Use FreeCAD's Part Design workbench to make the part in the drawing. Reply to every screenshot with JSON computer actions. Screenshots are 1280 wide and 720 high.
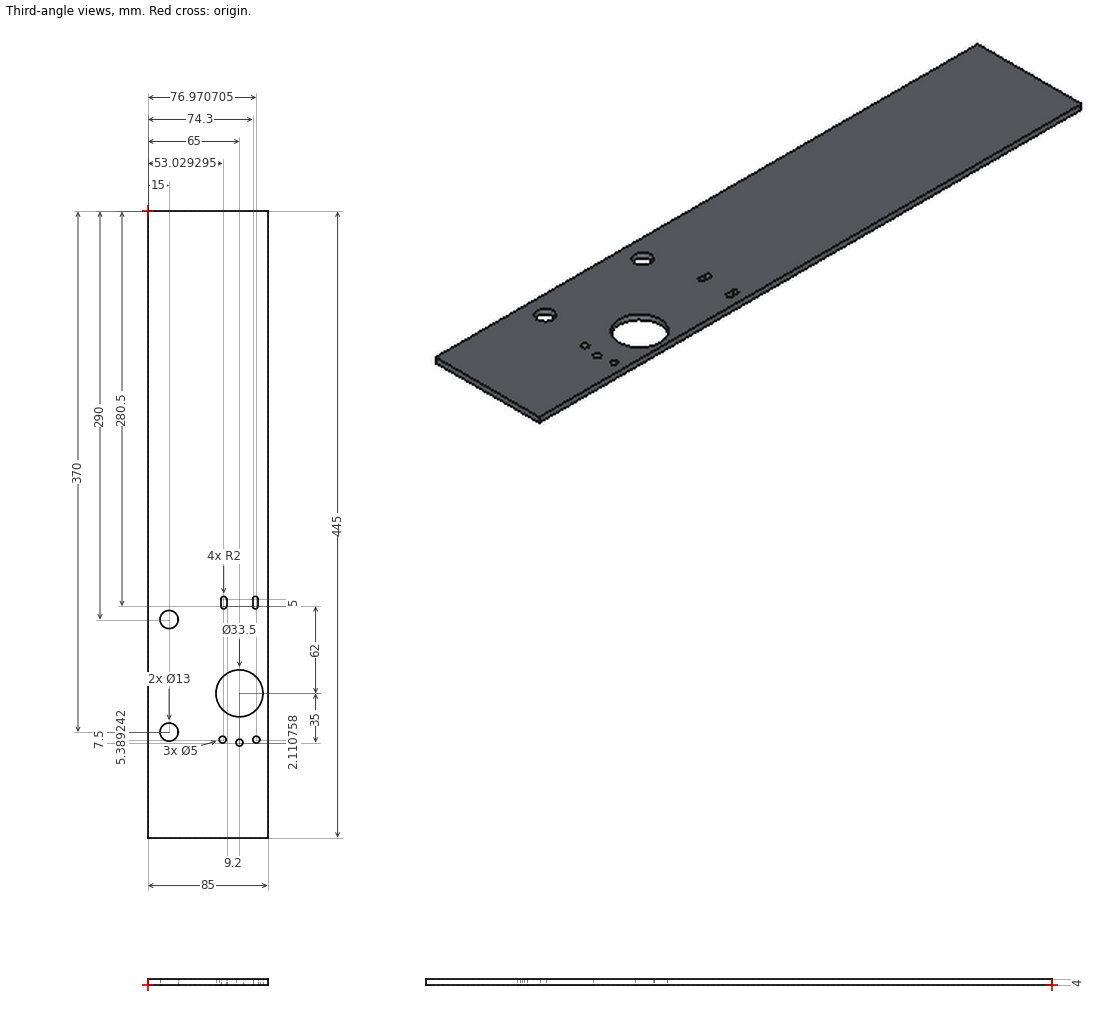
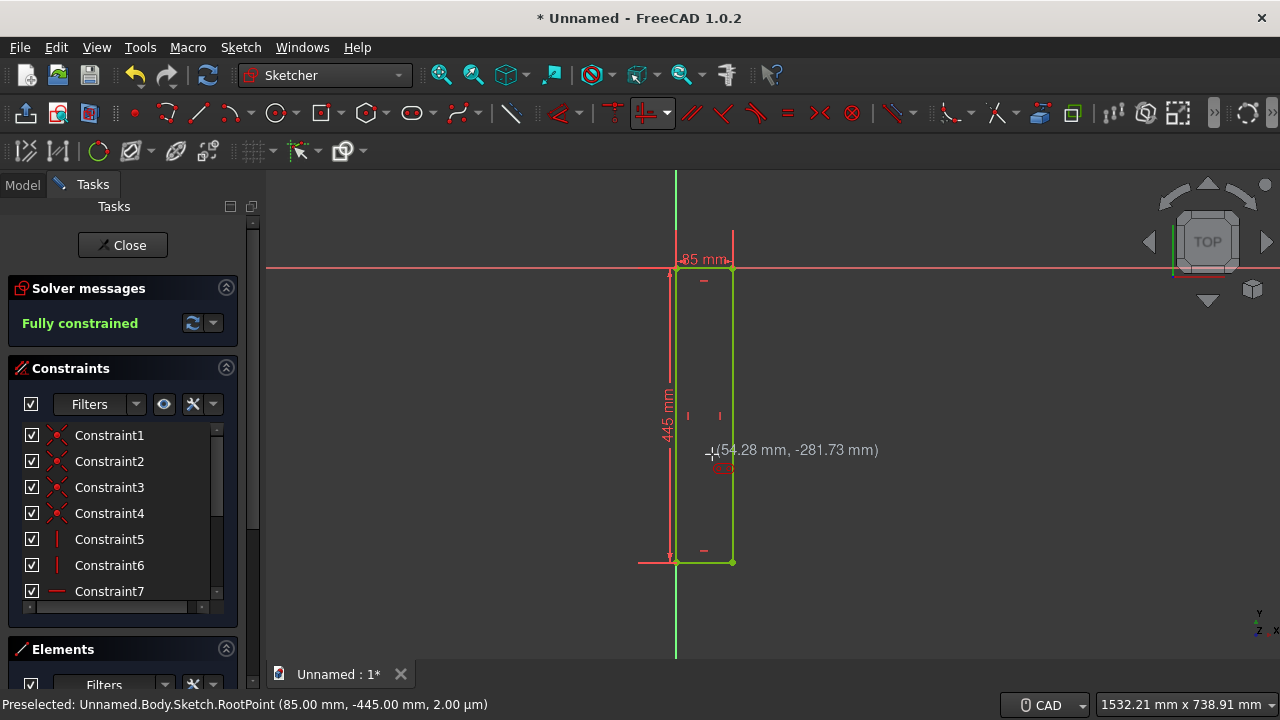
{"action": "left_click", "coordinate": [712, 454]}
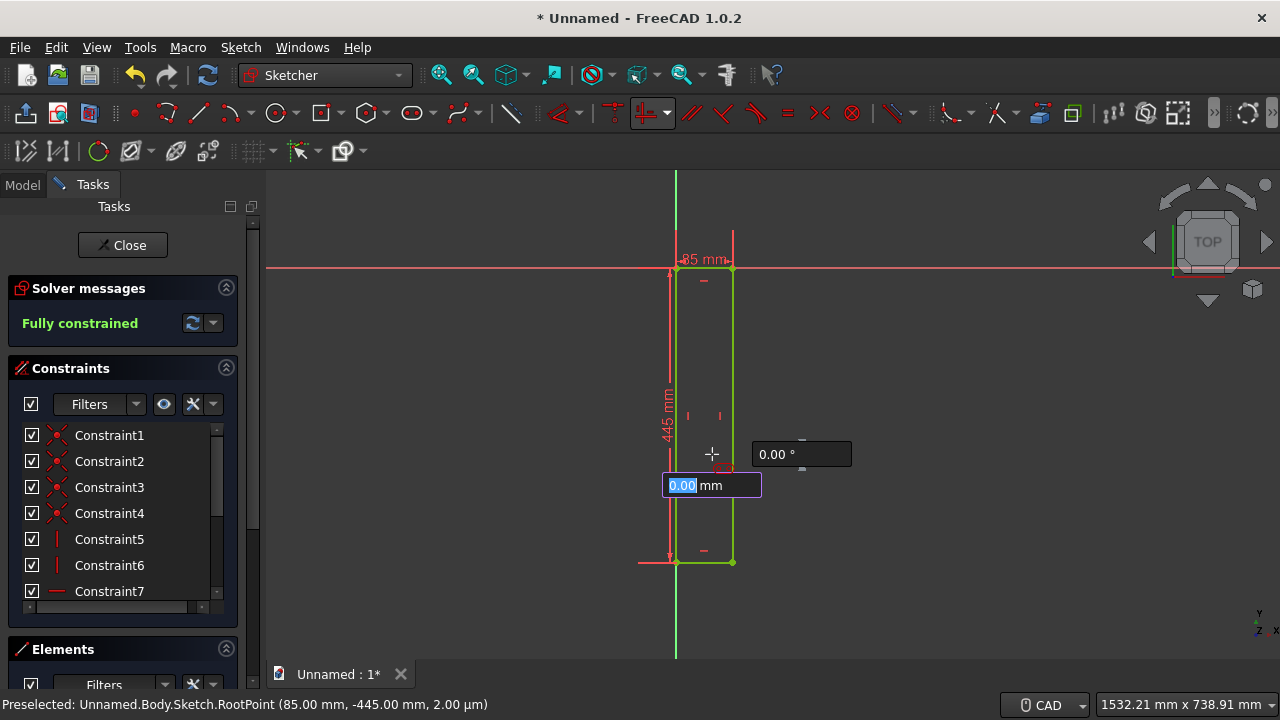
{"action": "scroll", "coordinate": [712, 450], "scroll_direction": "up", "scroll_amount": 8}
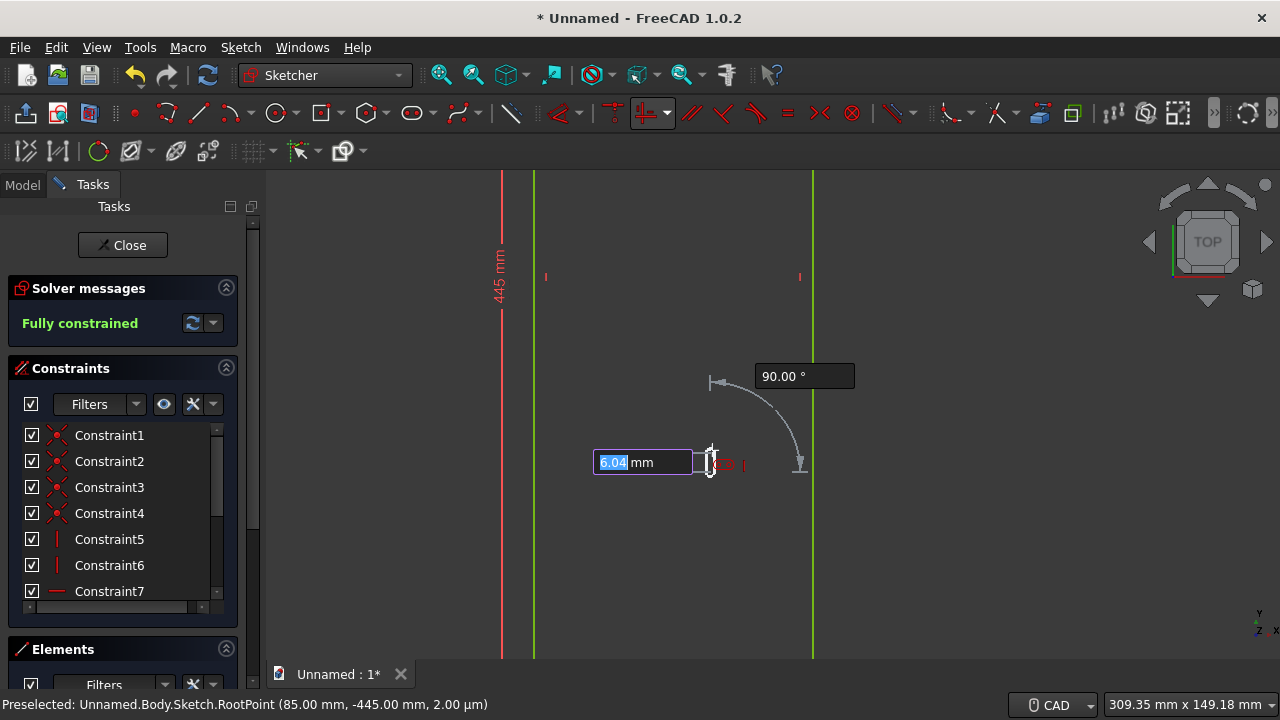
{"action": "left_click", "coordinate": [710, 450]}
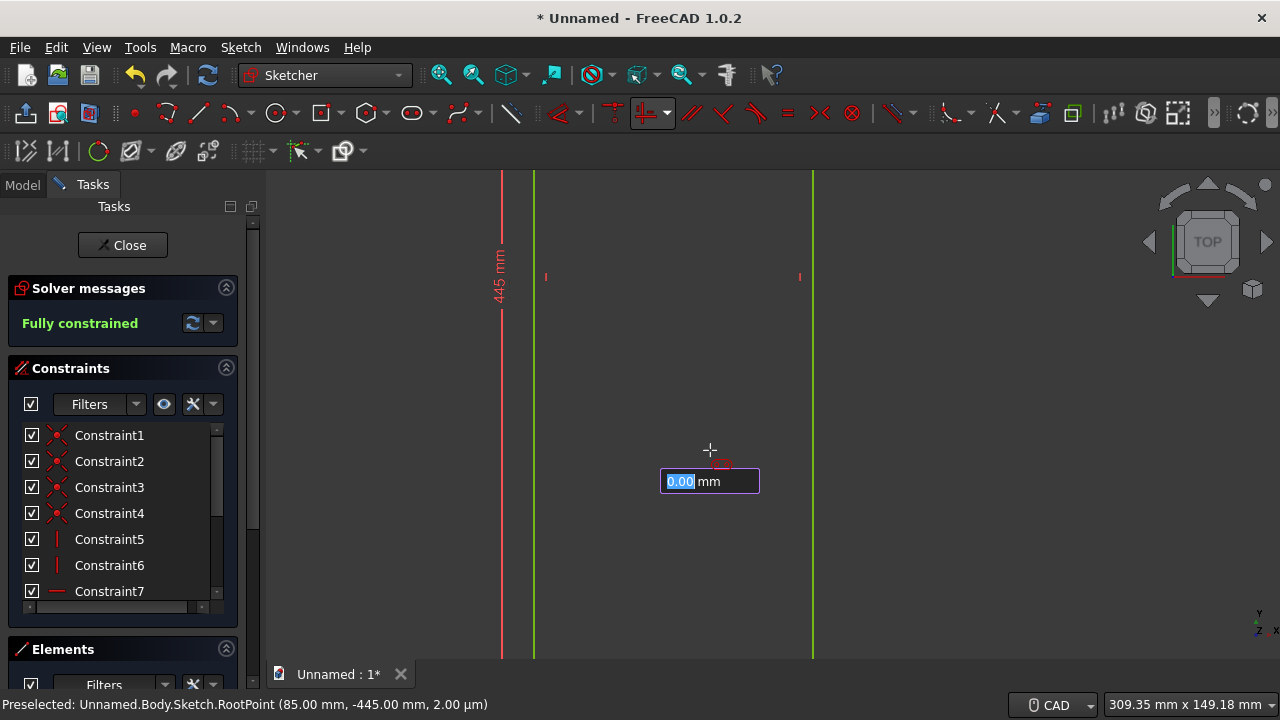
{"action": "scroll", "coordinate": [717, 458], "scroll_direction": "up", "scroll_amount": 5}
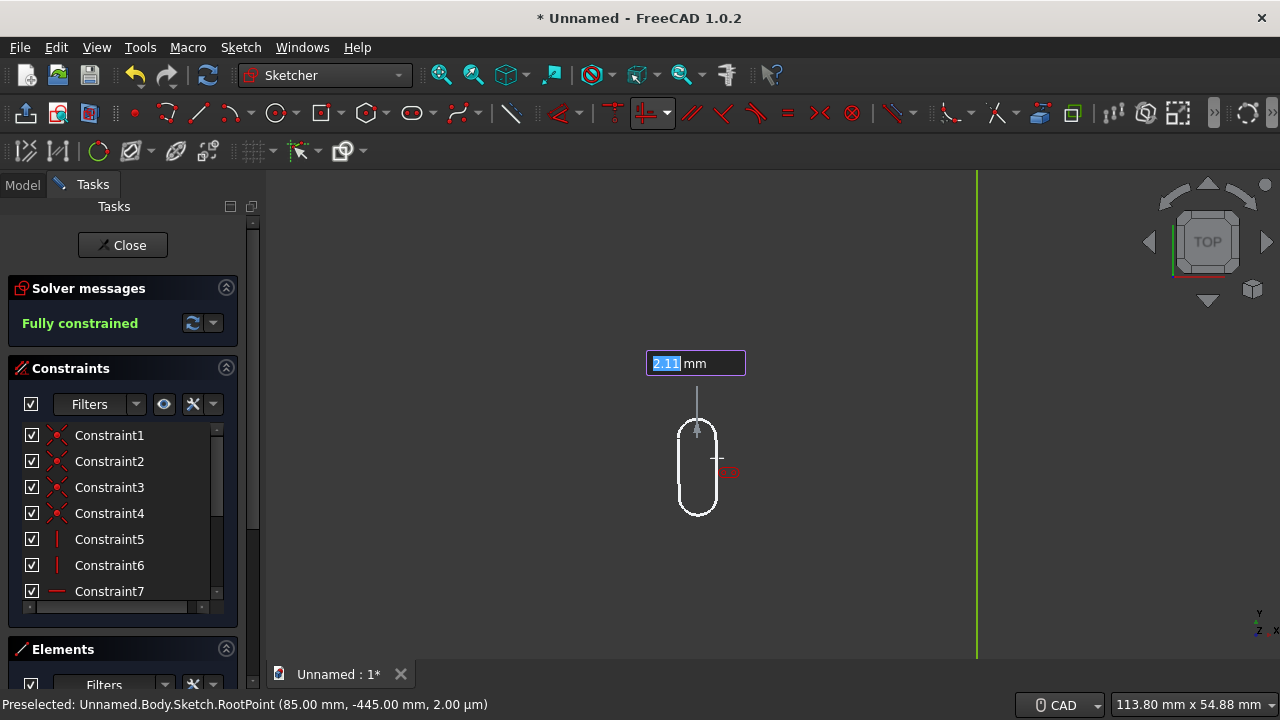
{"action": "left_click", "coordinate": [717, 458]}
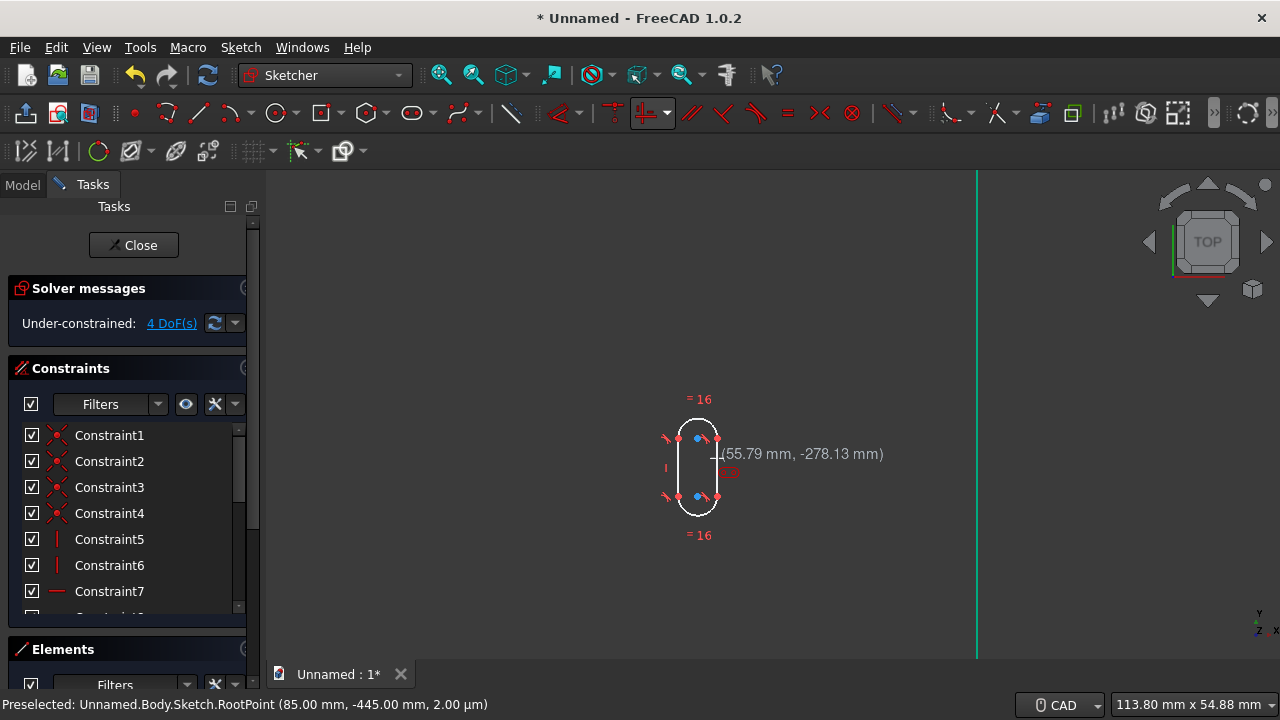
{"action": "scroll", "coordinate": [900, 480], "scroll_direction": "up", "scroll_amount": 2}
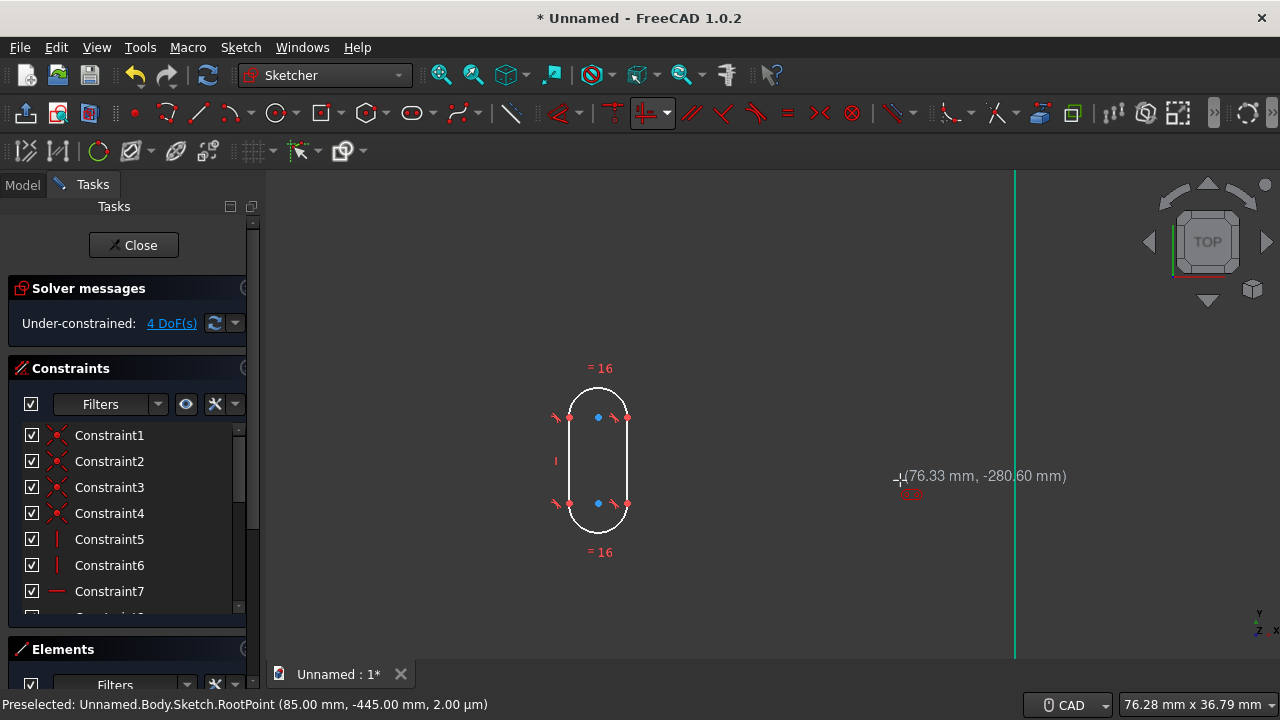
{"action": "scroll", "coordinate": [718, 451], "scroll_direction": "down", "scroll_amount": 15}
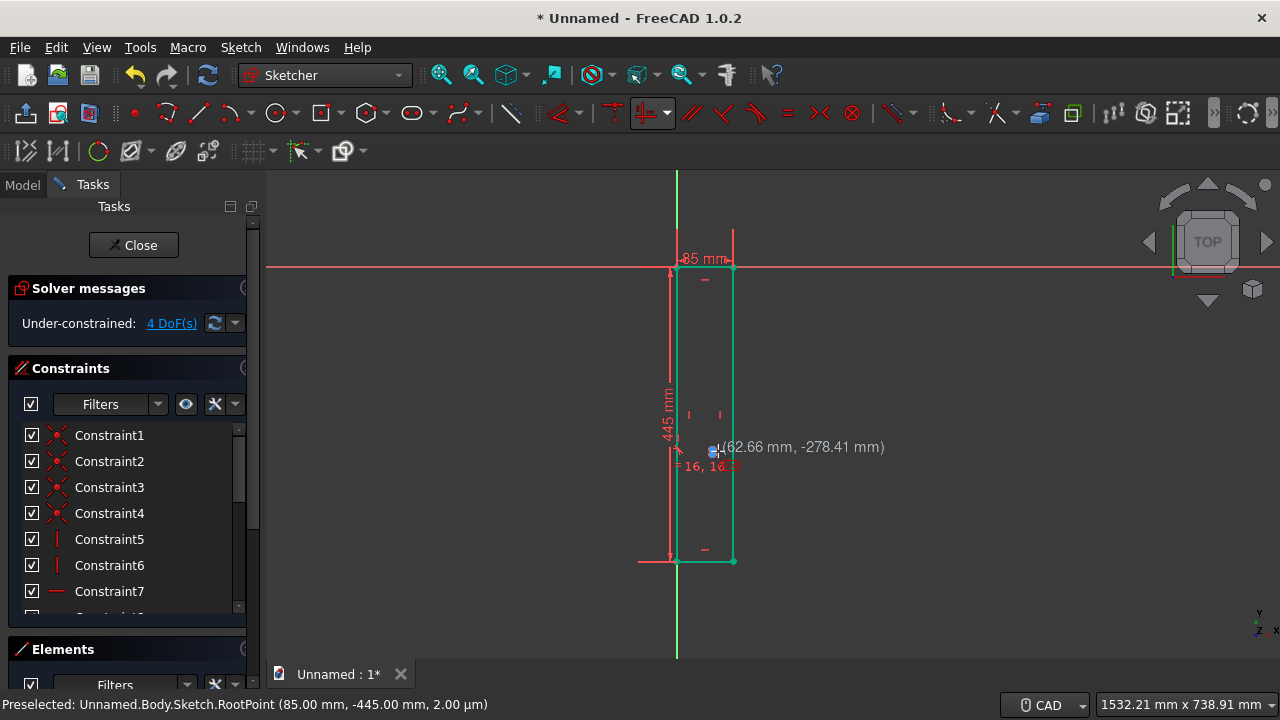
{"action": "scroll", "coordinate": [727, 453], "scroll_direction": "up", "scroll_amount": 6}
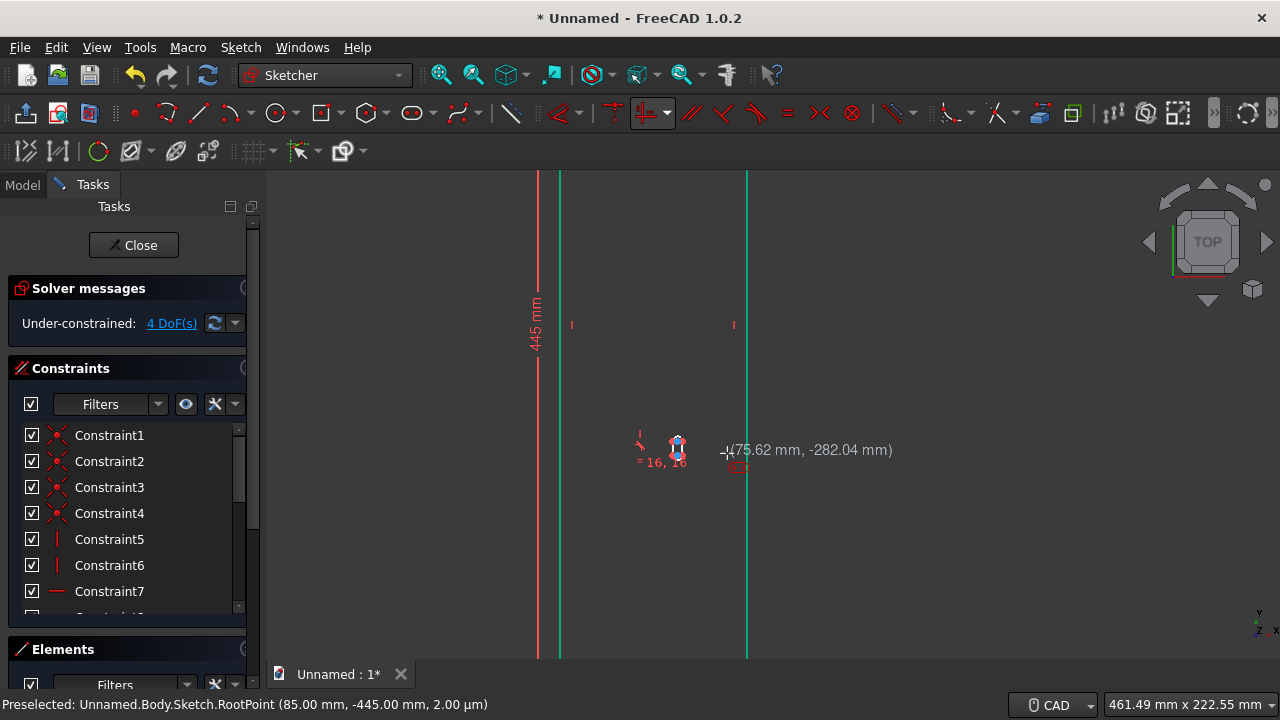
{"action": "left_click", "coordinate": [727, 452]}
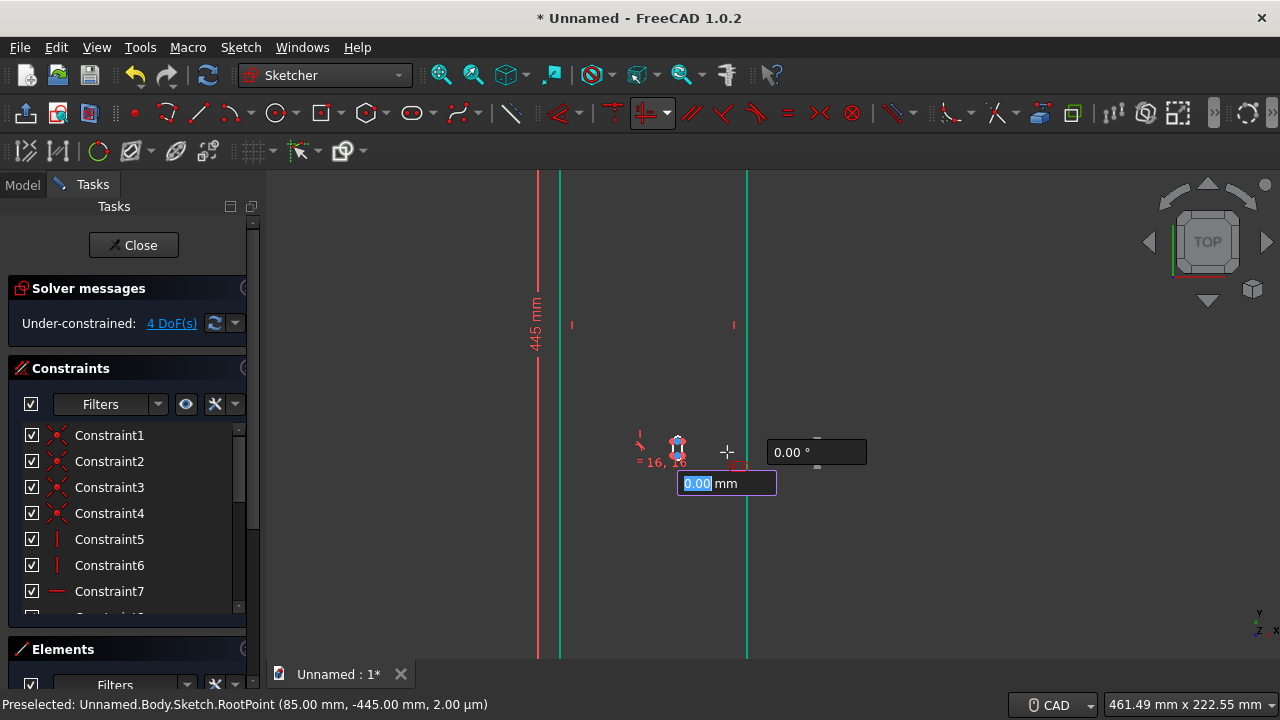
{"action": "scroll", "coordinate": [727, 441], "scroll_direction": "up", "scroll_amount": 2}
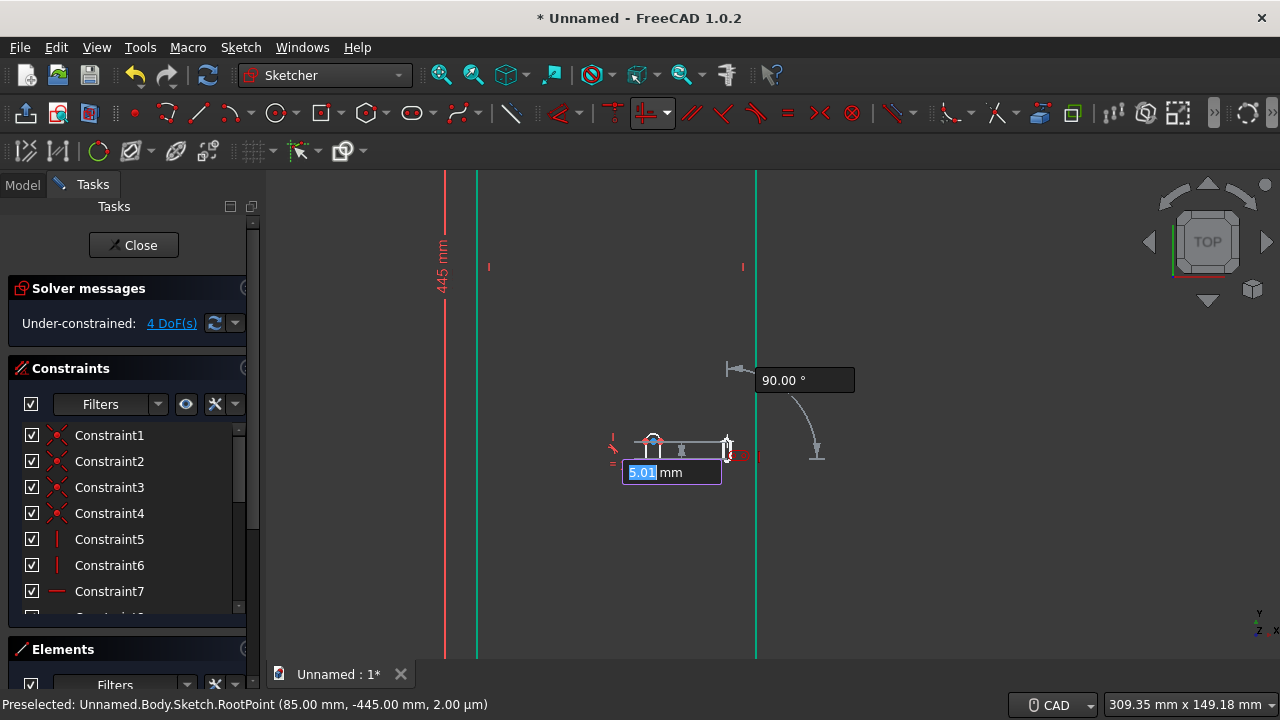
{"action": "left_click", "coordinate": [727, 440]}